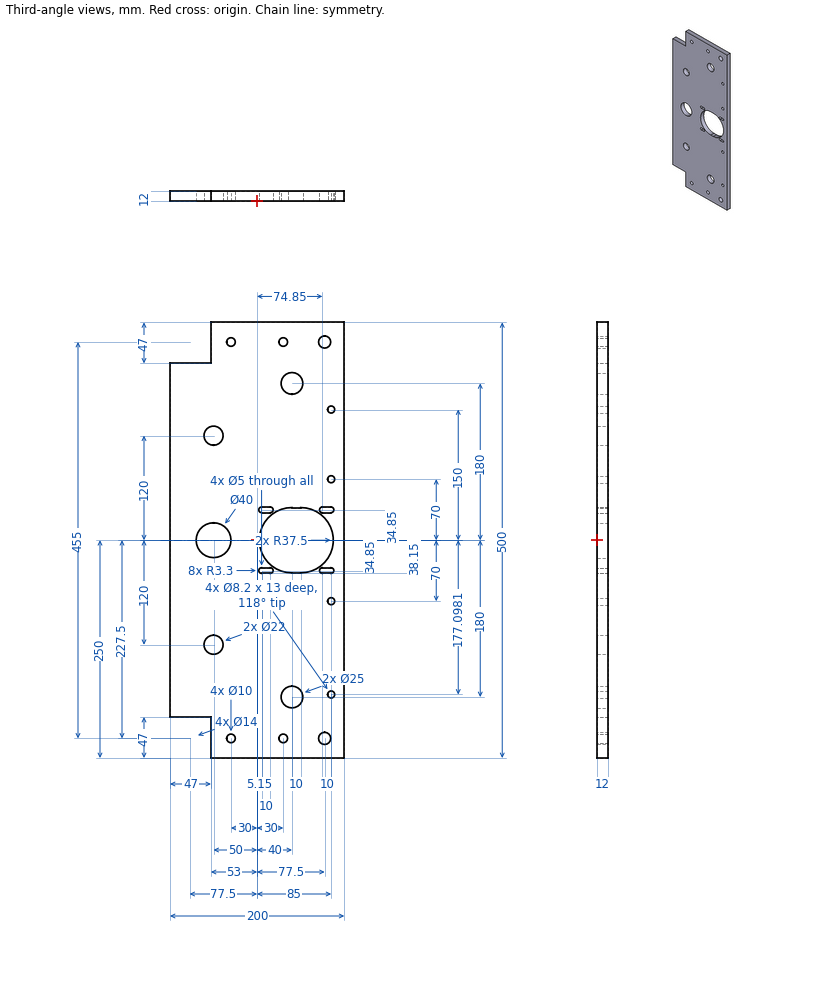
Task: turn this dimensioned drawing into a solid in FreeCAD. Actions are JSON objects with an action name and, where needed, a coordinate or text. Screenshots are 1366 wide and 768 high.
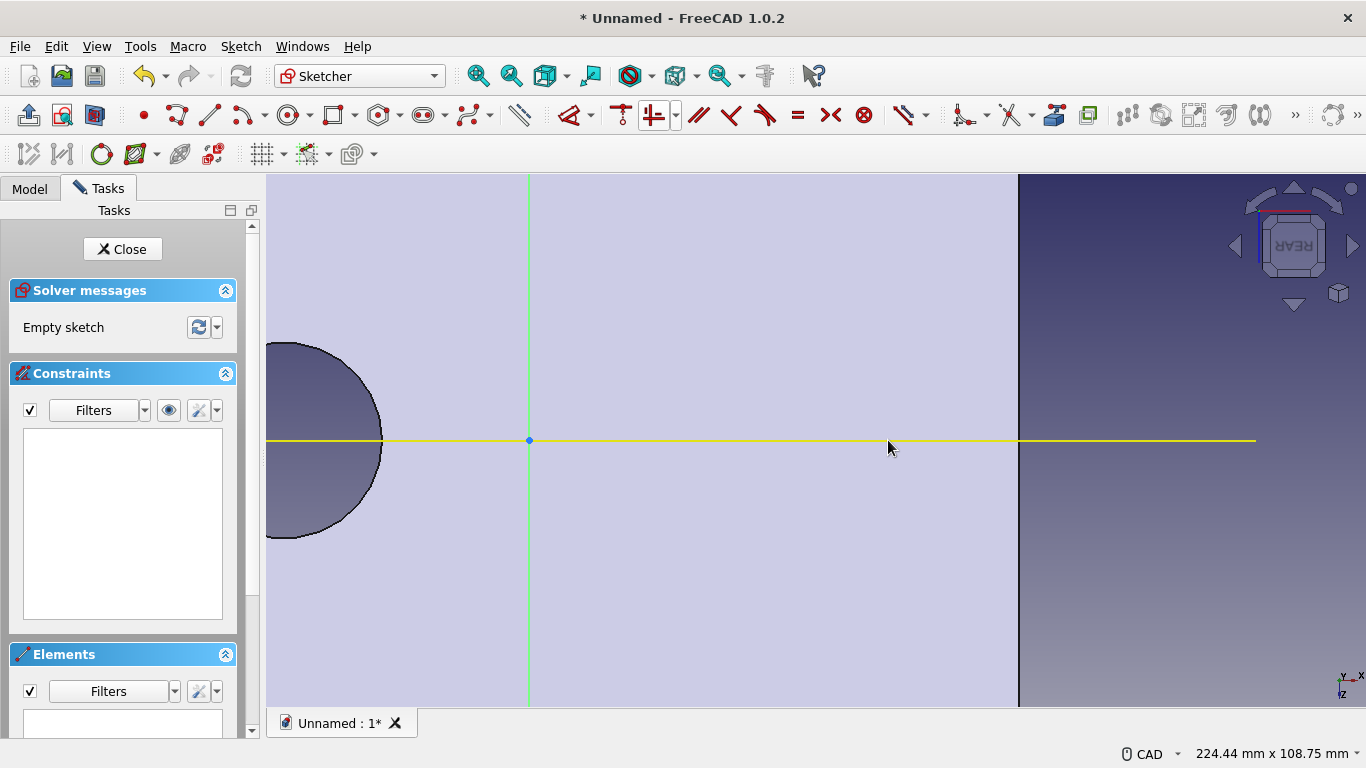
{"action": "key", "text": "g s"}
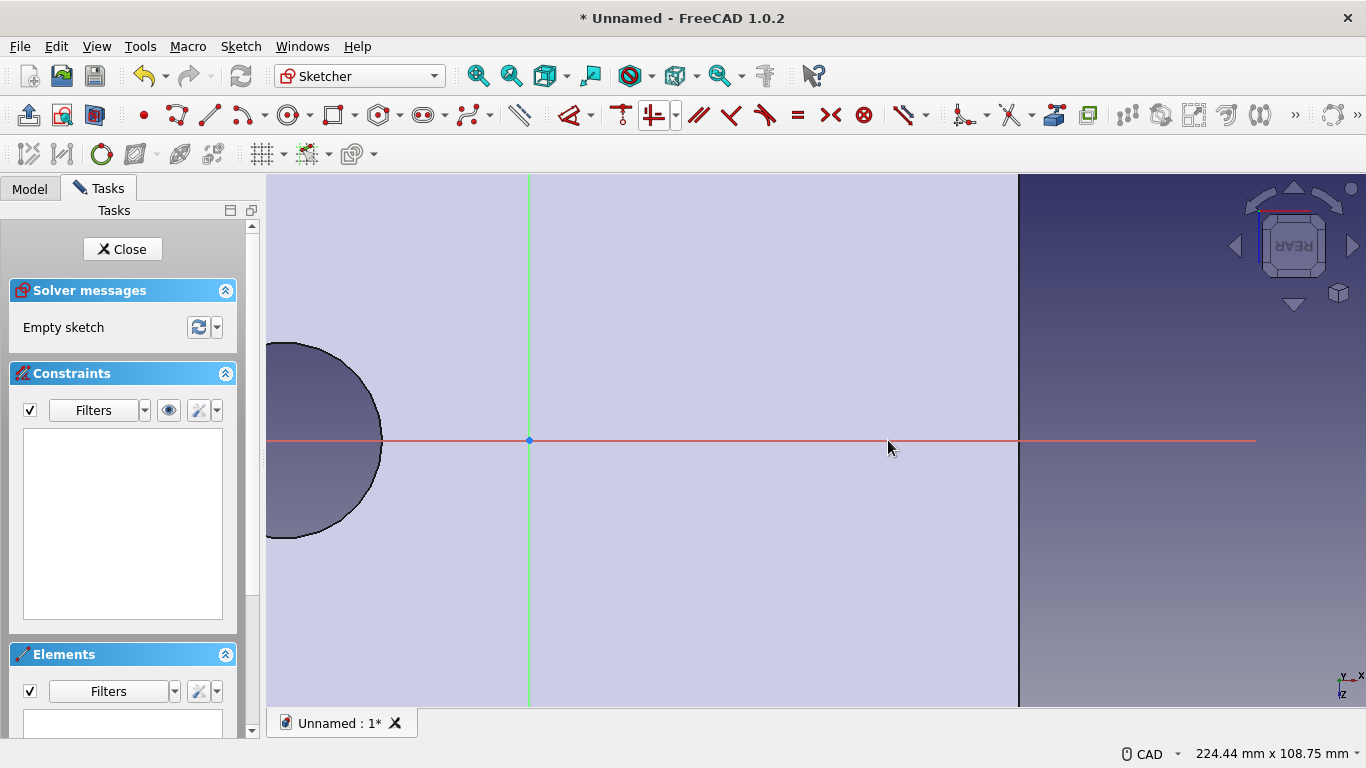
{"action": "left_click", "coordinate": [725, 440]}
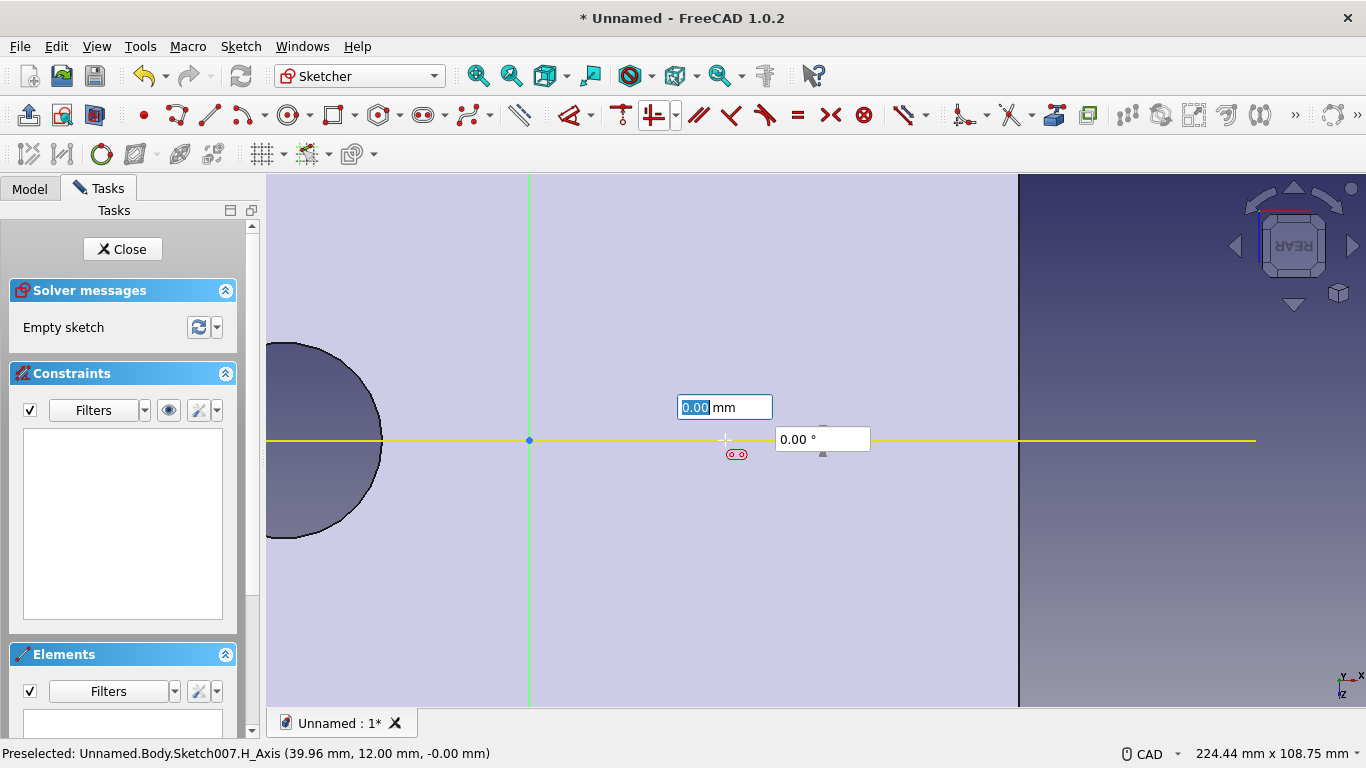
{"action": "left_click", "coordinate": [774, 431]}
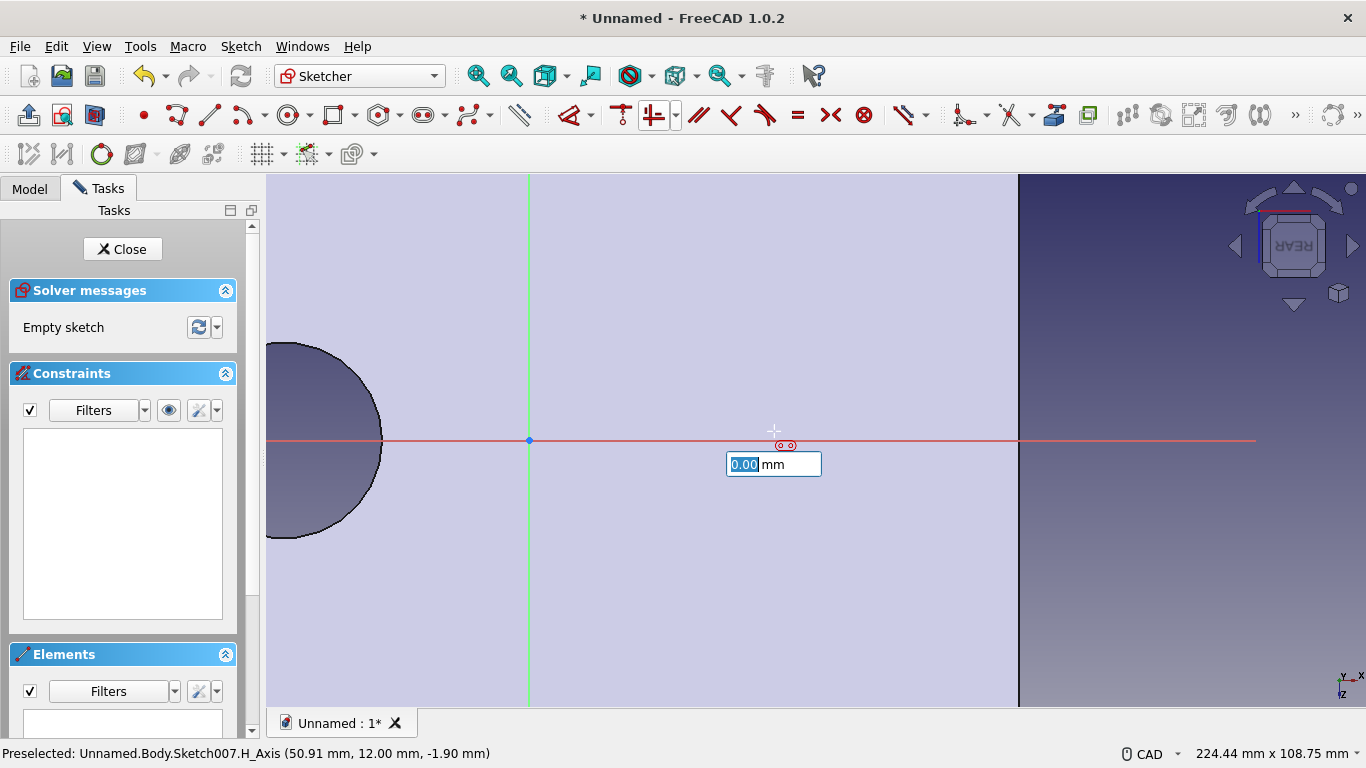
{"action": "left_click", "coordinate": [750, 624]}
{"action": "key", "text": "Escape"}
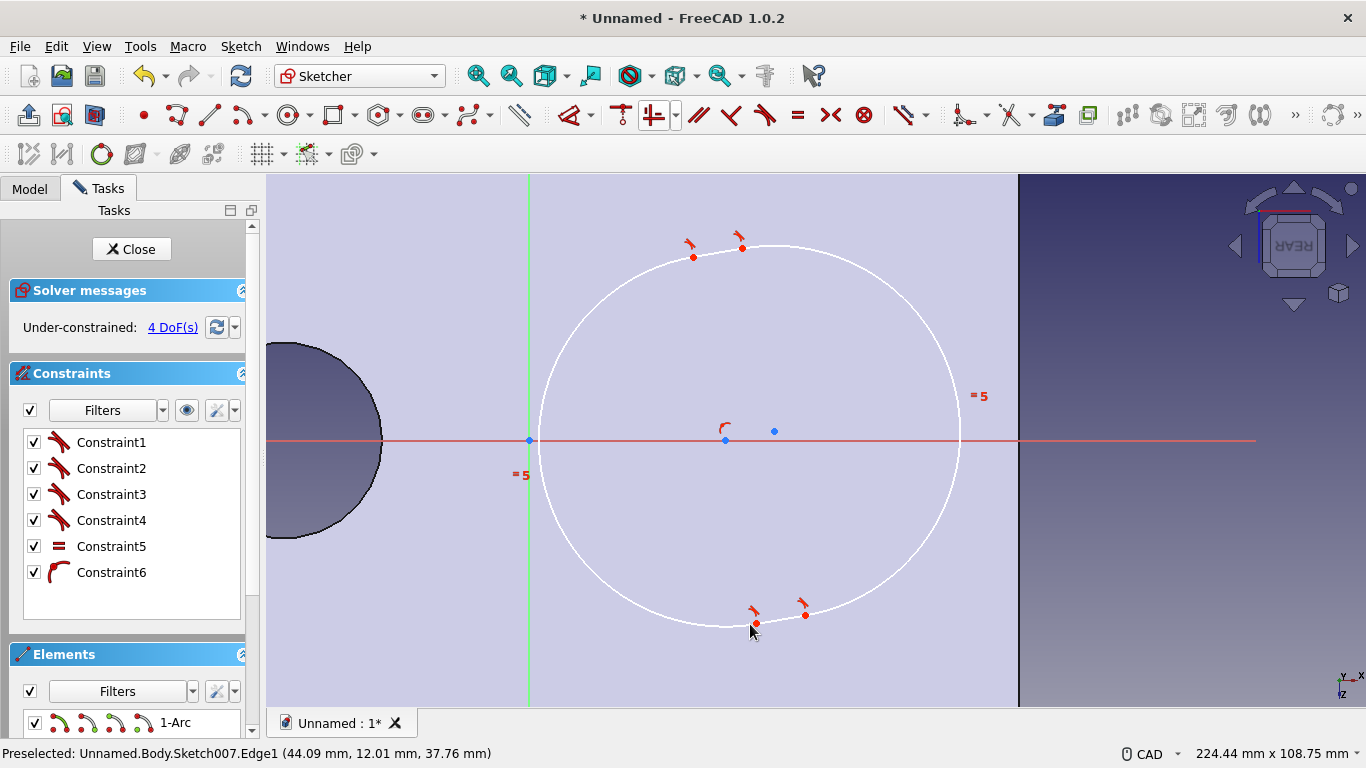
{"action": "key", "text": "d"}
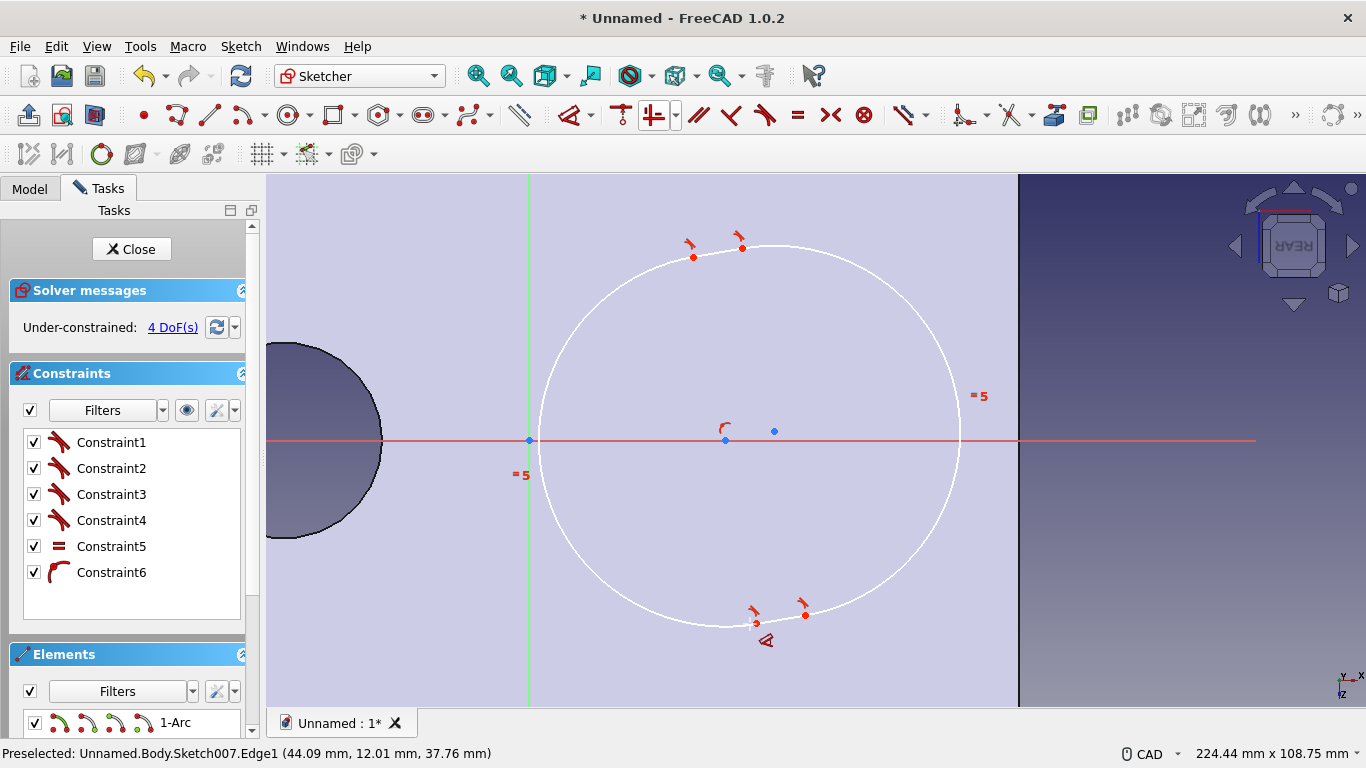
{"action": "left_click", "coordinate": [558, 358]}
{"action": "left_click", "coordinate": [600, 262]}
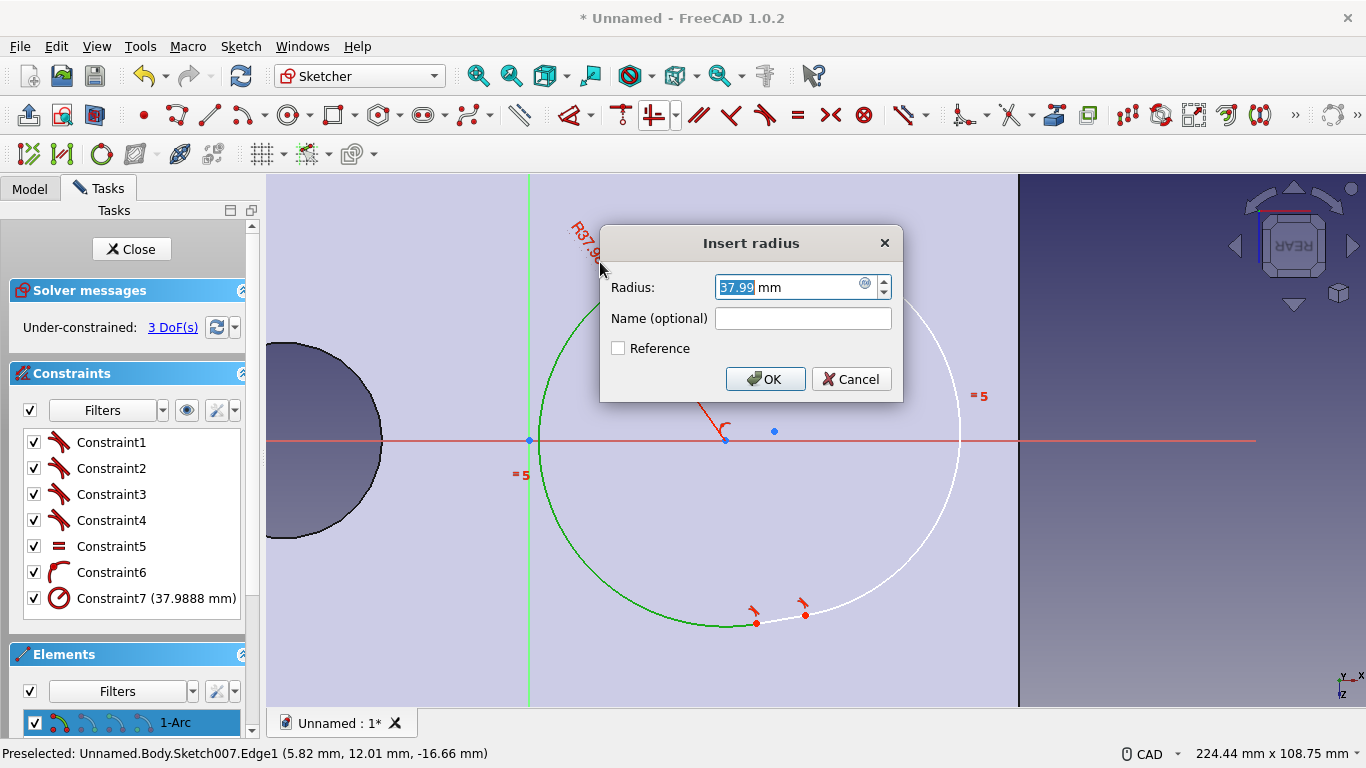
{"action": "type", "text": "37.5"}
{"action": "key", "text": "Return"}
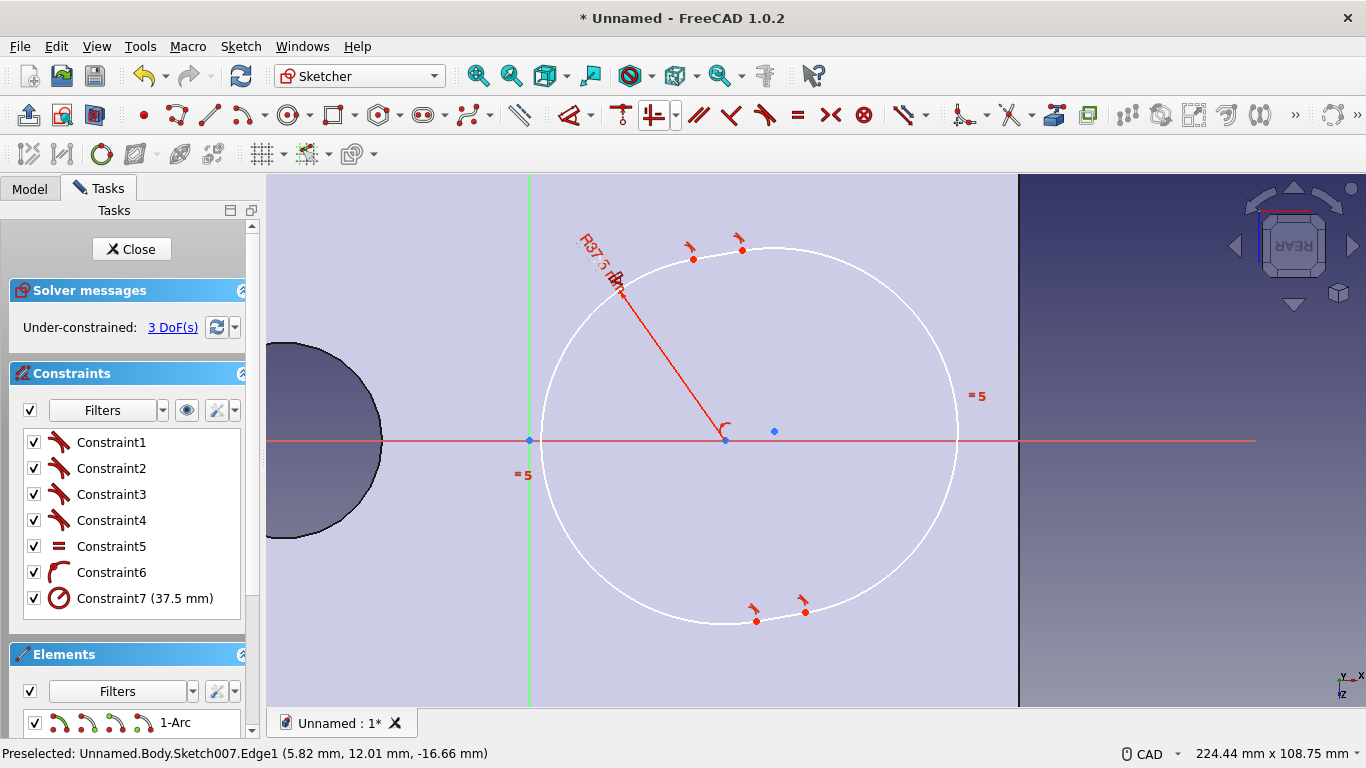
{"action": "left_click", "coordinate": [708, 257]}
{"action": "left_click", "coordinate": [718, 217]}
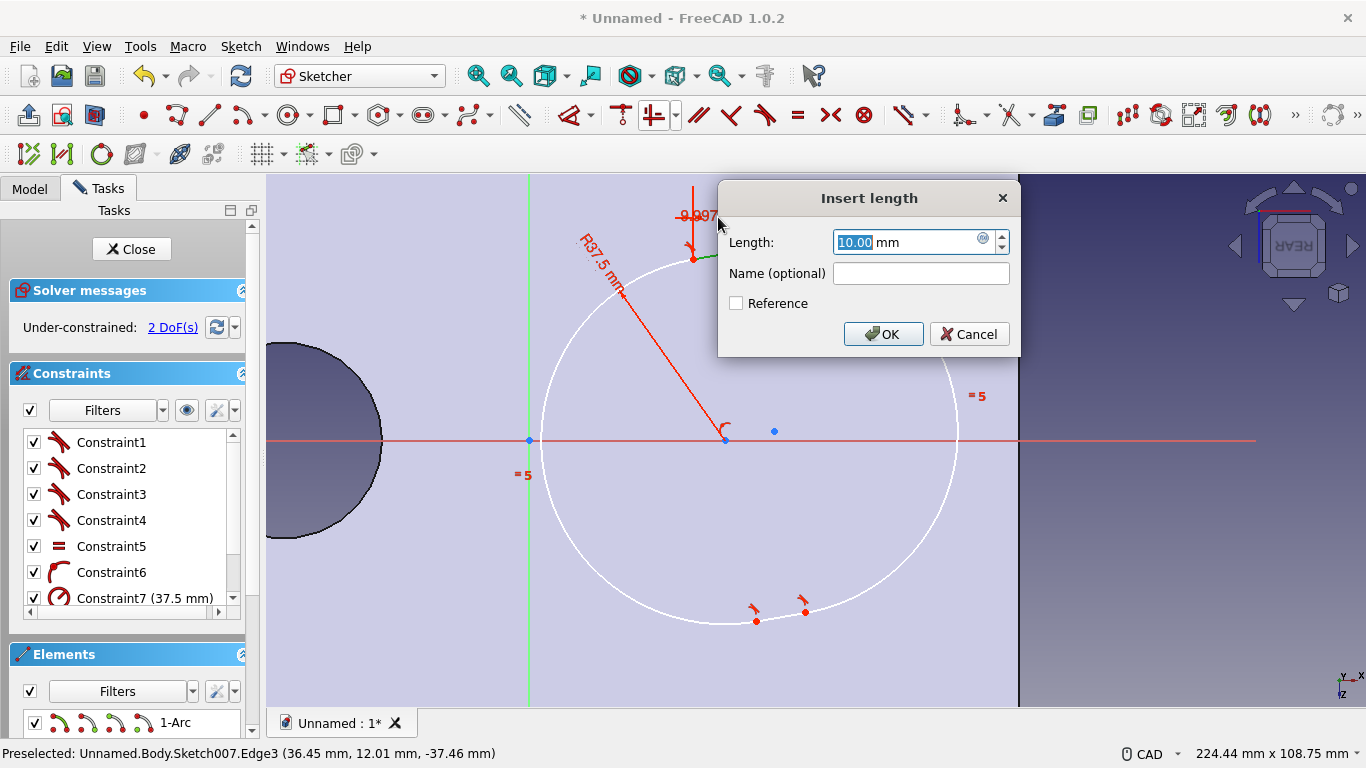
{"action": "type", "text": "10"}
{"action": "key", "text": "Return"}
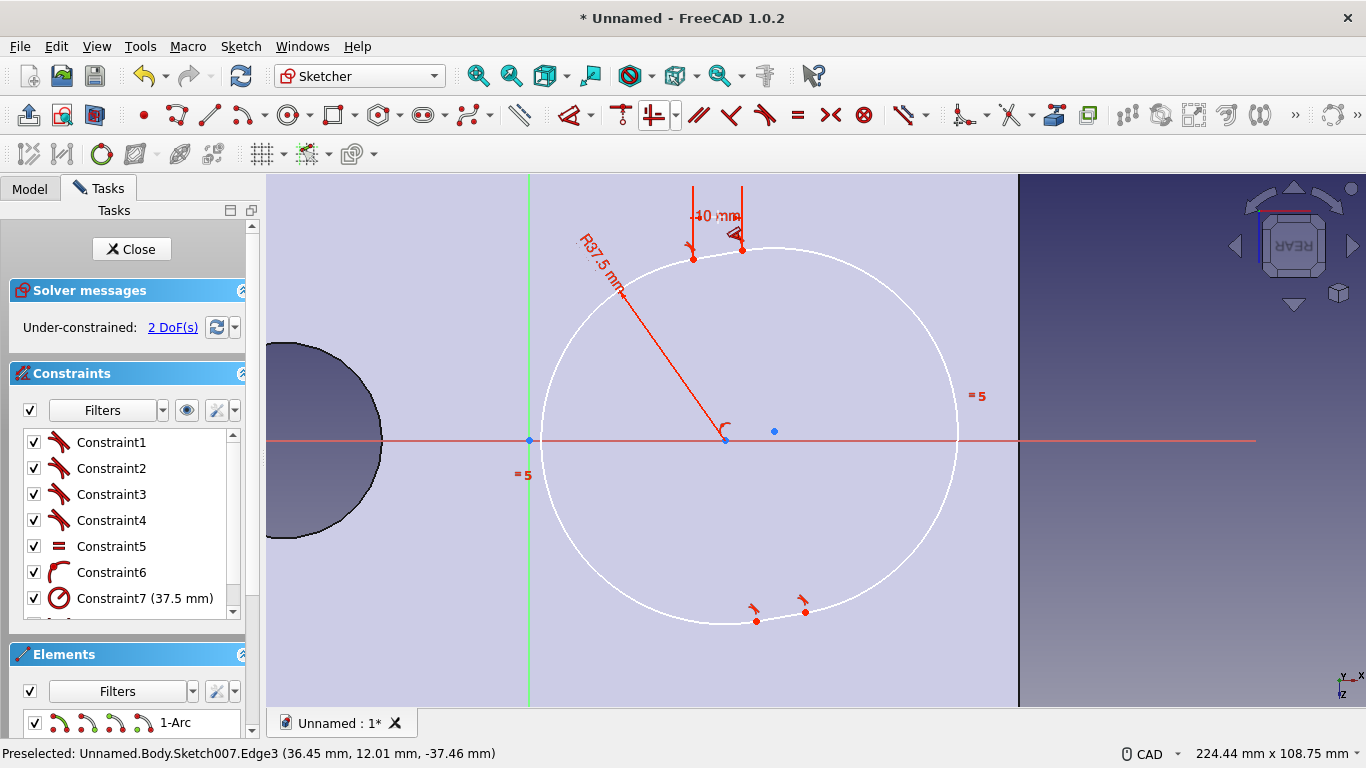
{"action": "left_click", "coordinate": [693, 259]}
{"action": "left_click", "coordinate": [611, 225]}